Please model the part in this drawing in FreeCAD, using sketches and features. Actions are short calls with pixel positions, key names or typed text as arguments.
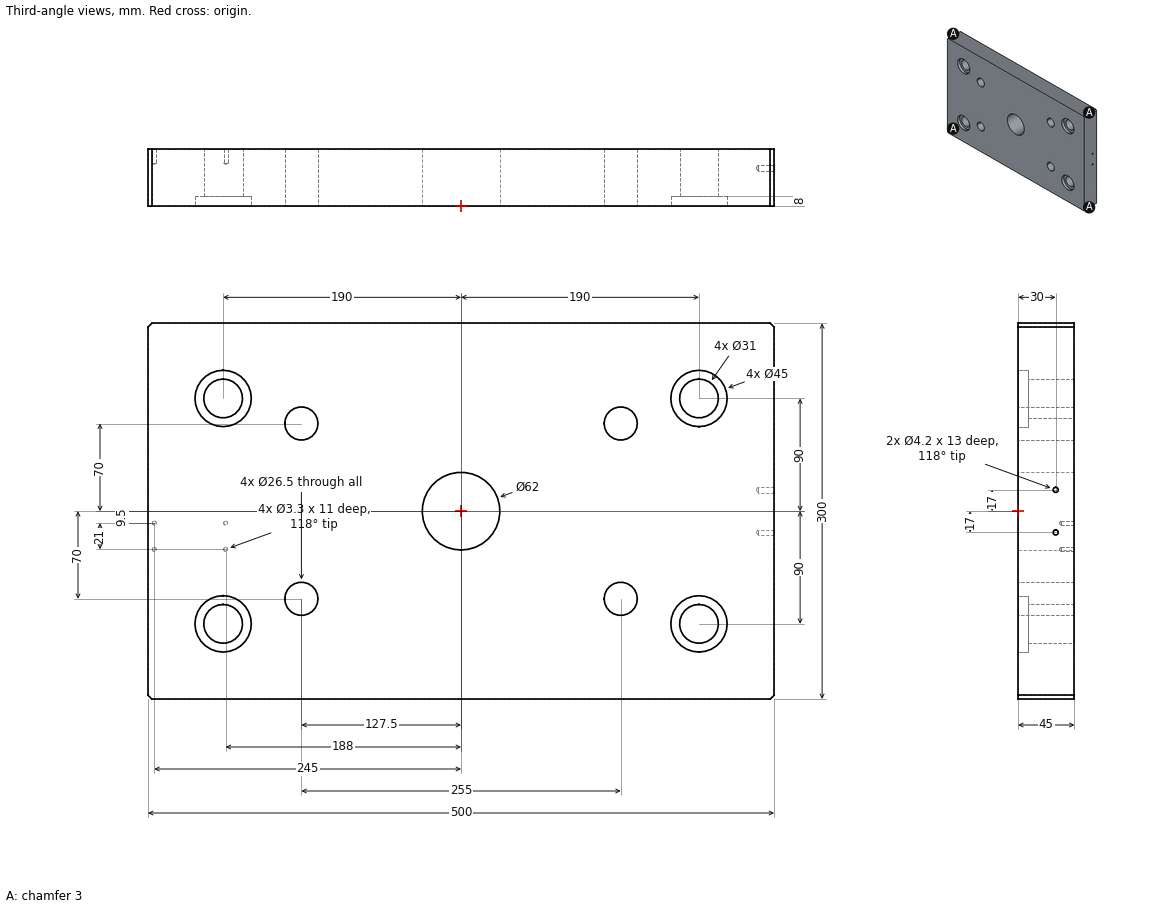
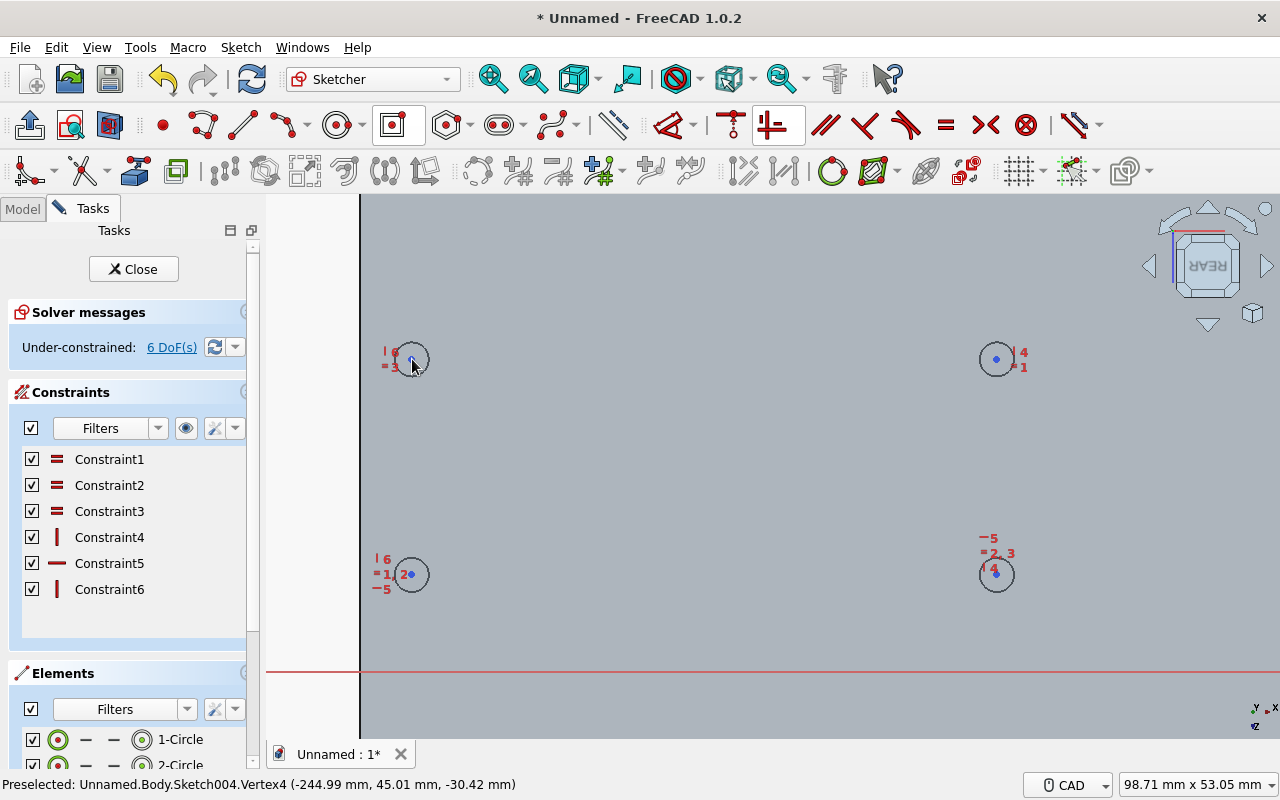
click(997, 359)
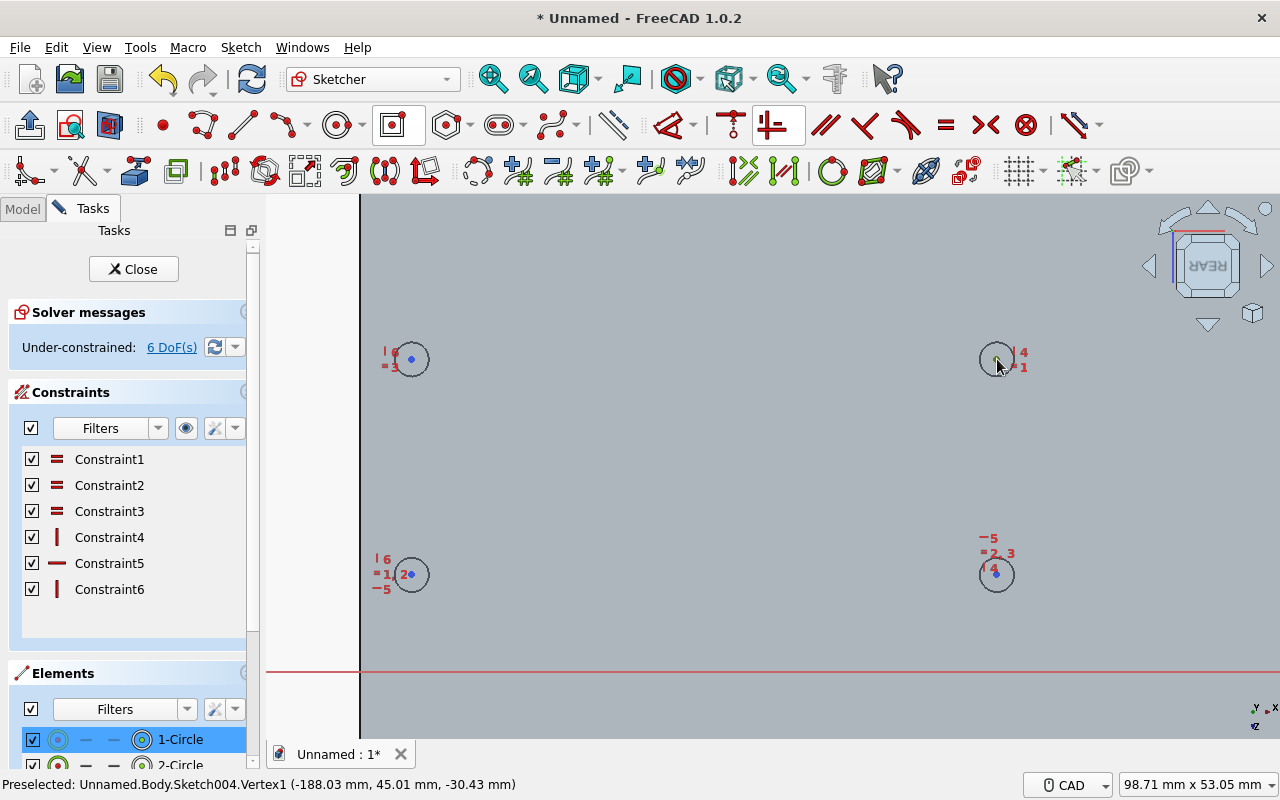
click(412, 359)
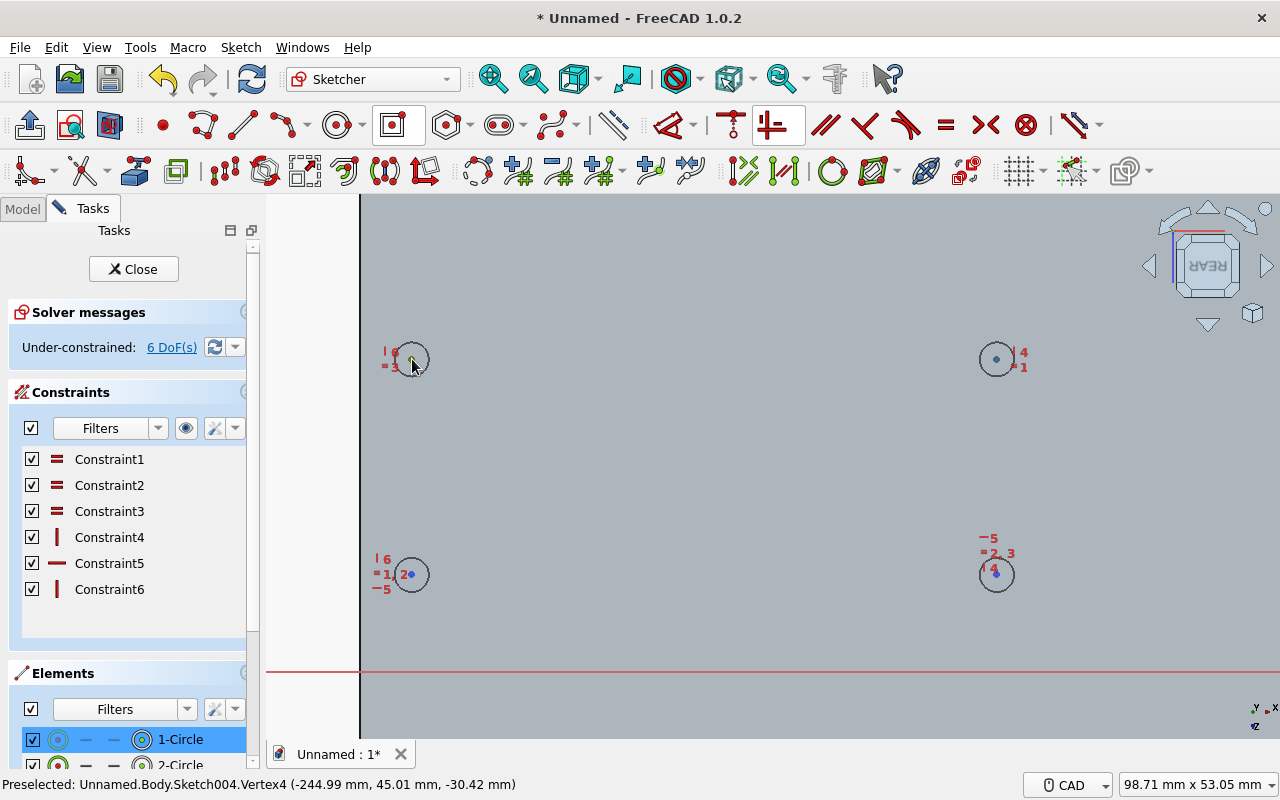
click(800, 126)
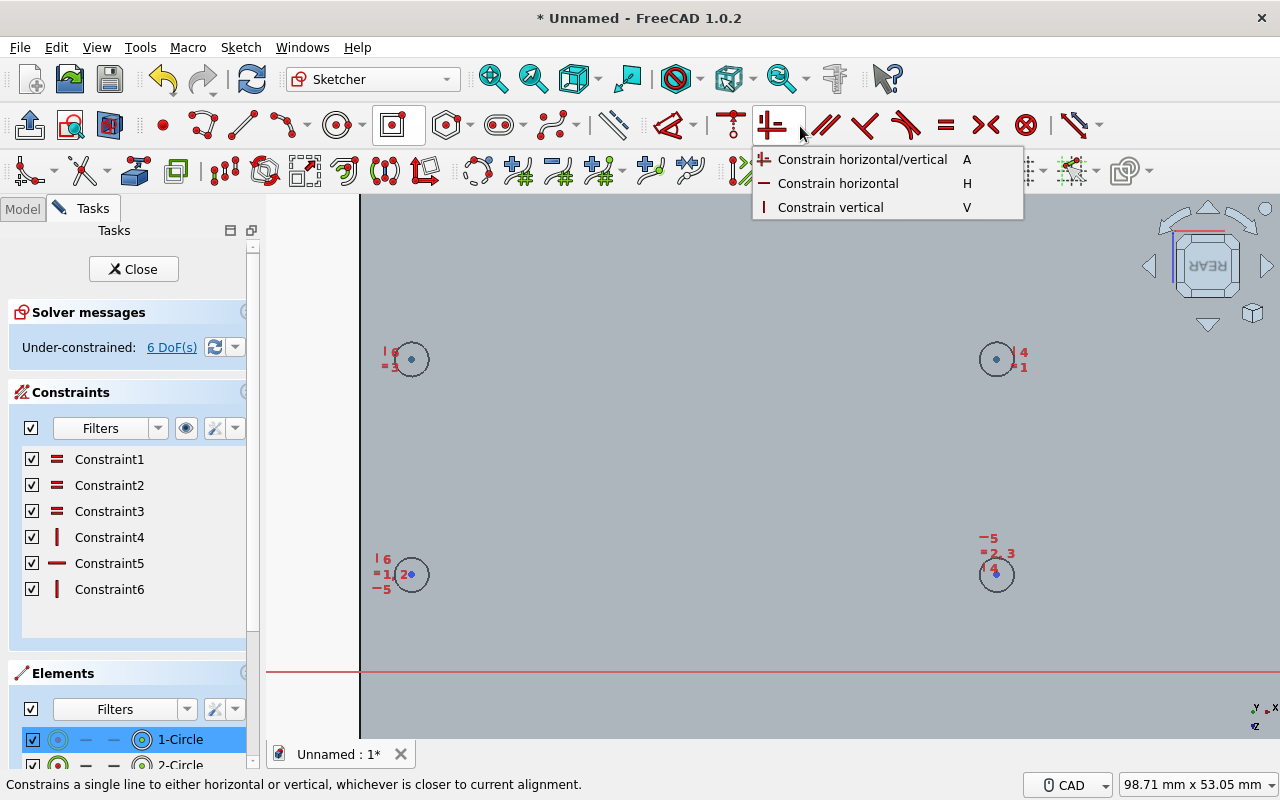
click(888, 183)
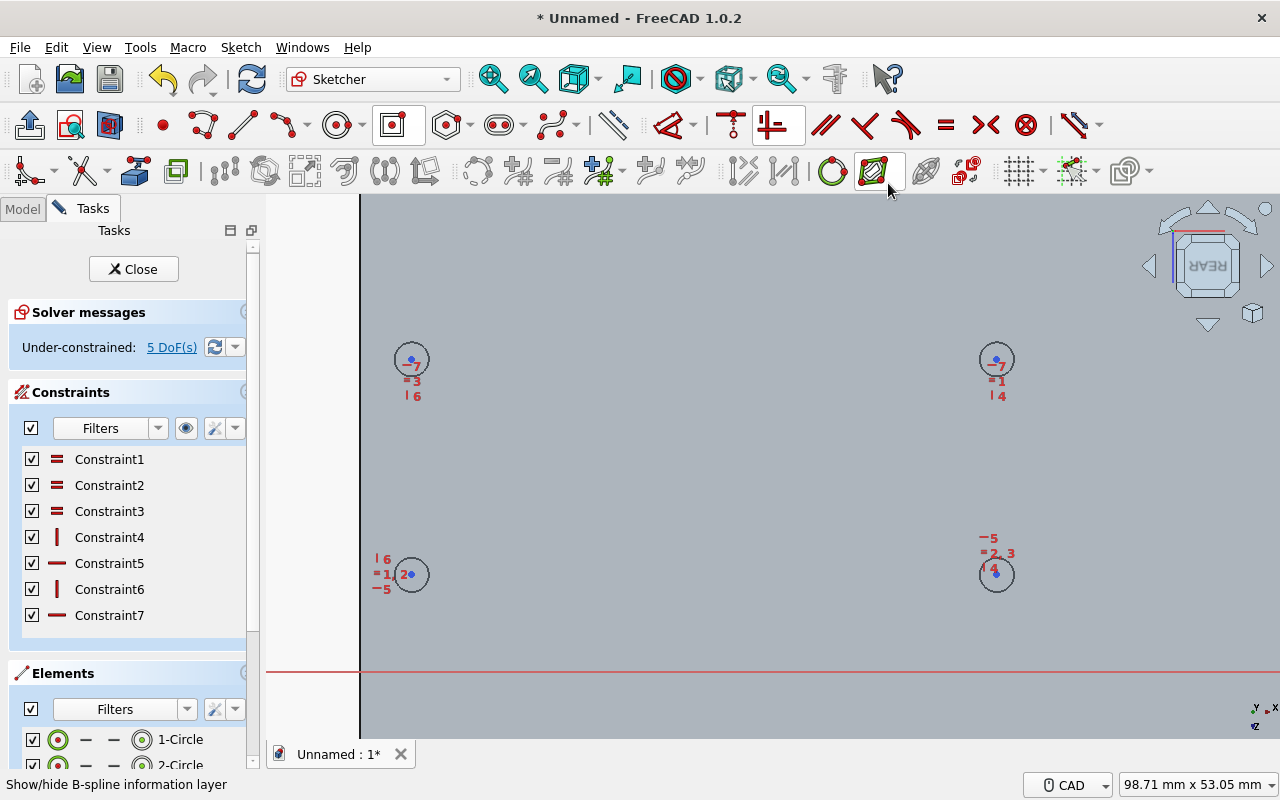
click(668, 126)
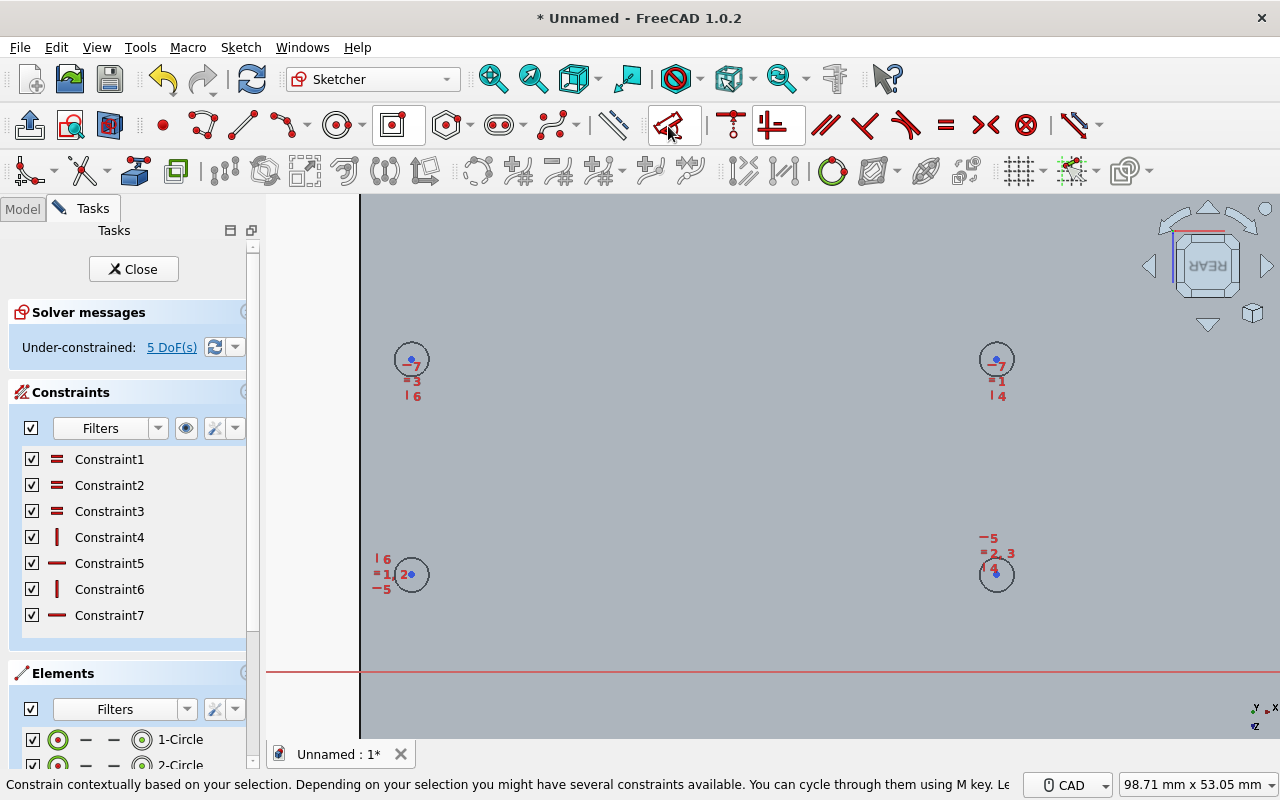
click(1009, 347)
click(1031, 324)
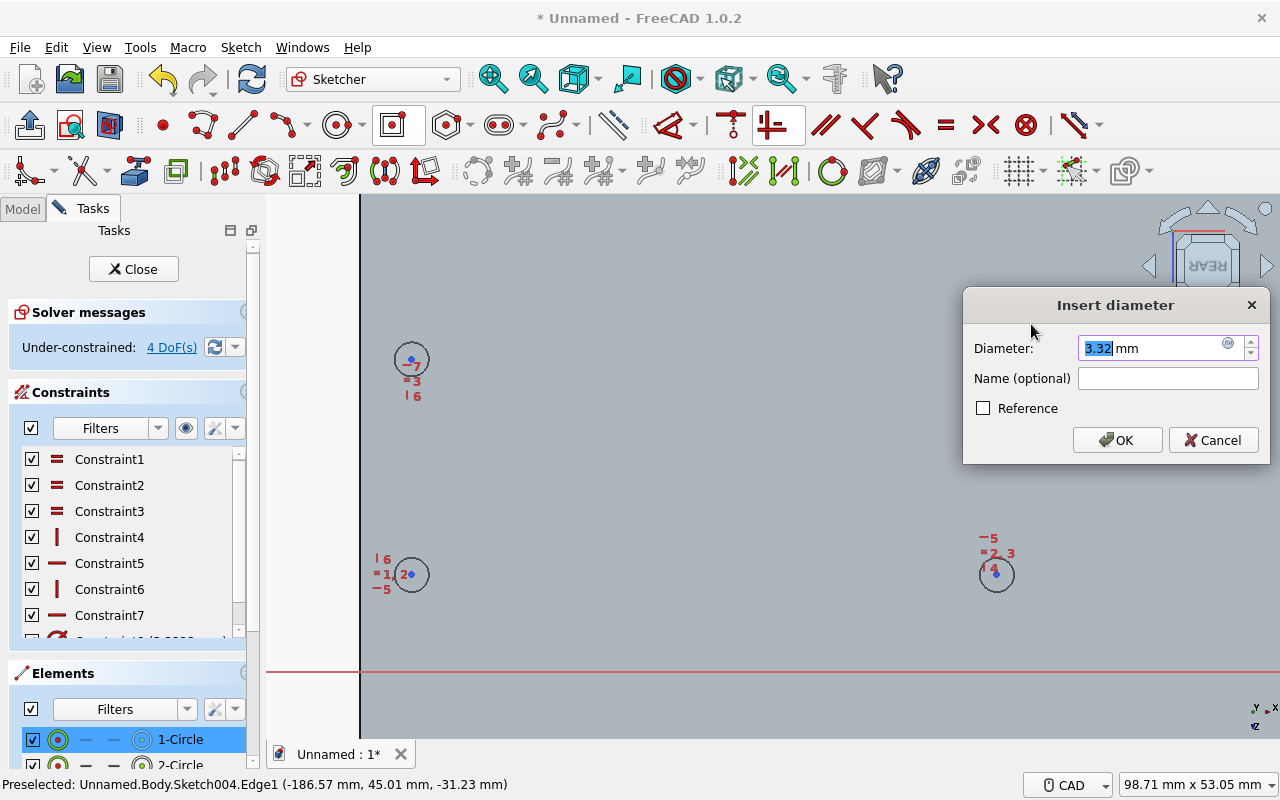
text(3.3)
key(Return)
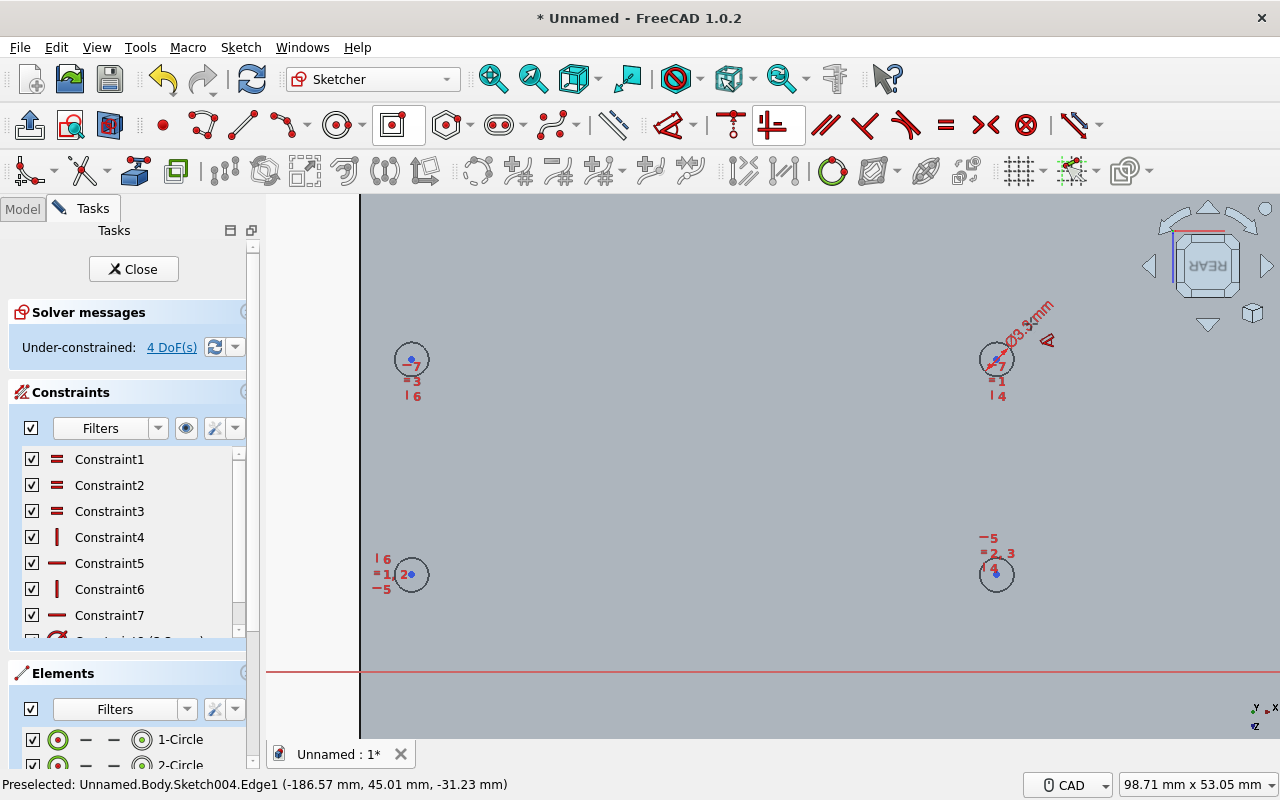
click(997, 359)
click(1056, 706)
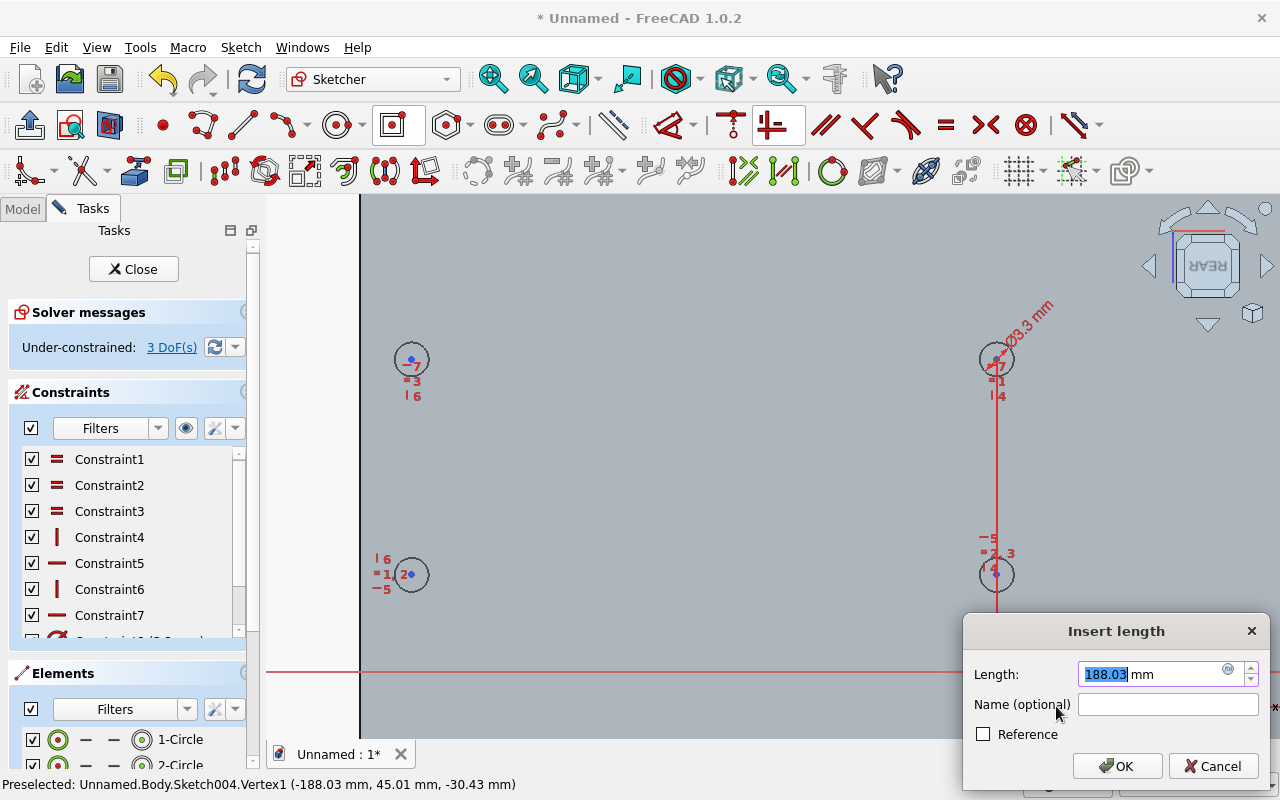
text(188)
key(Return)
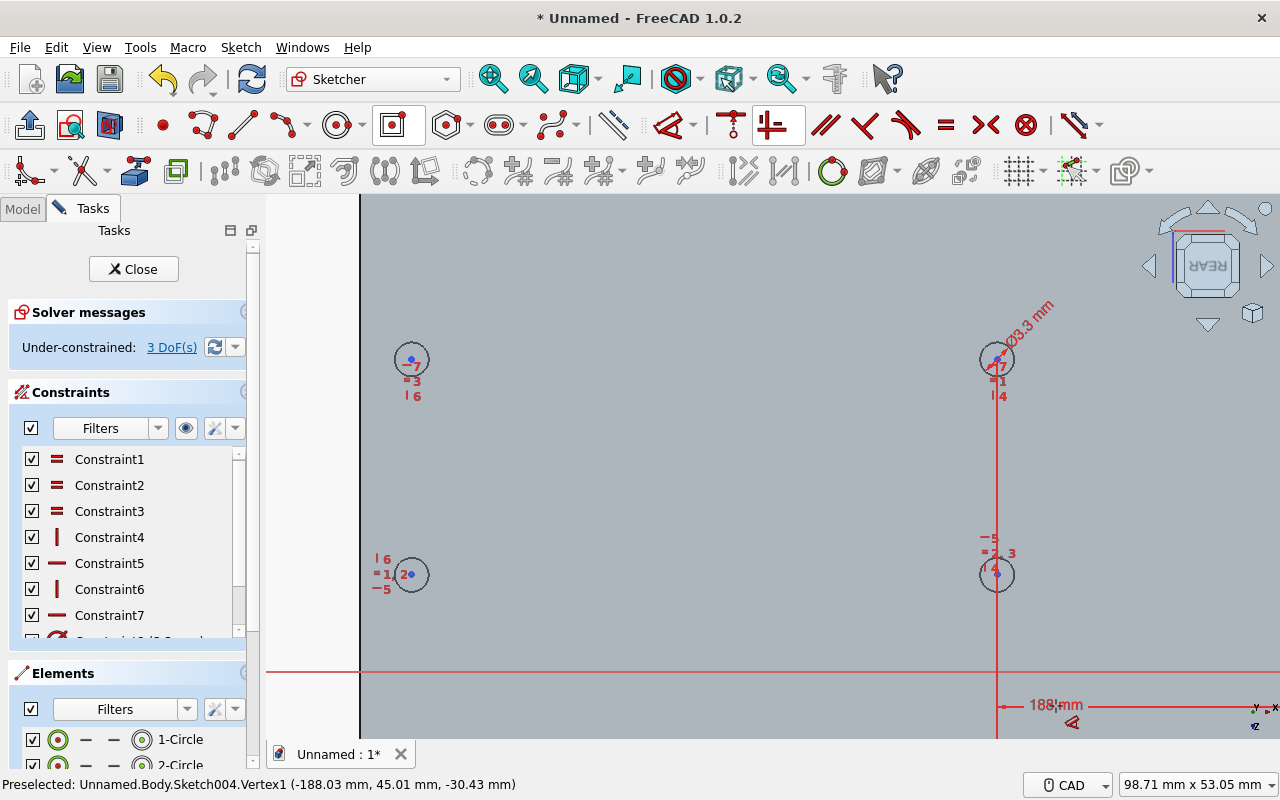
click(412, 575)
click(763, 706)